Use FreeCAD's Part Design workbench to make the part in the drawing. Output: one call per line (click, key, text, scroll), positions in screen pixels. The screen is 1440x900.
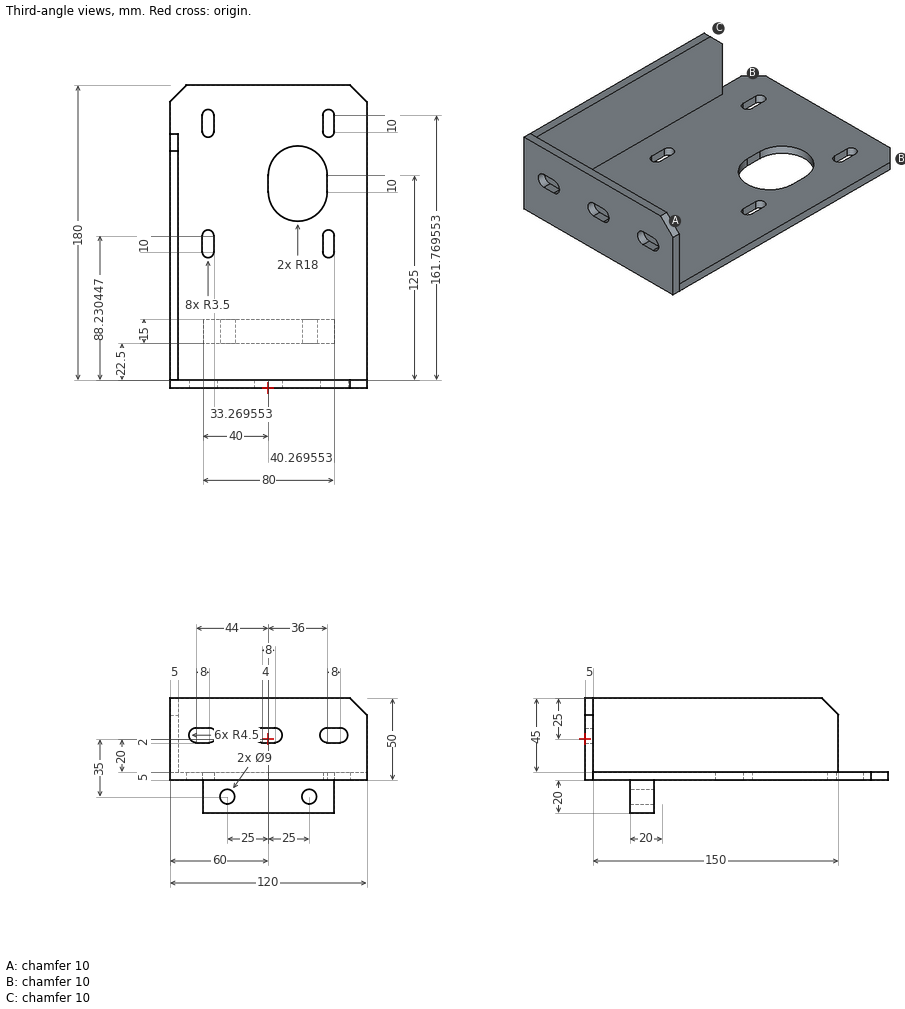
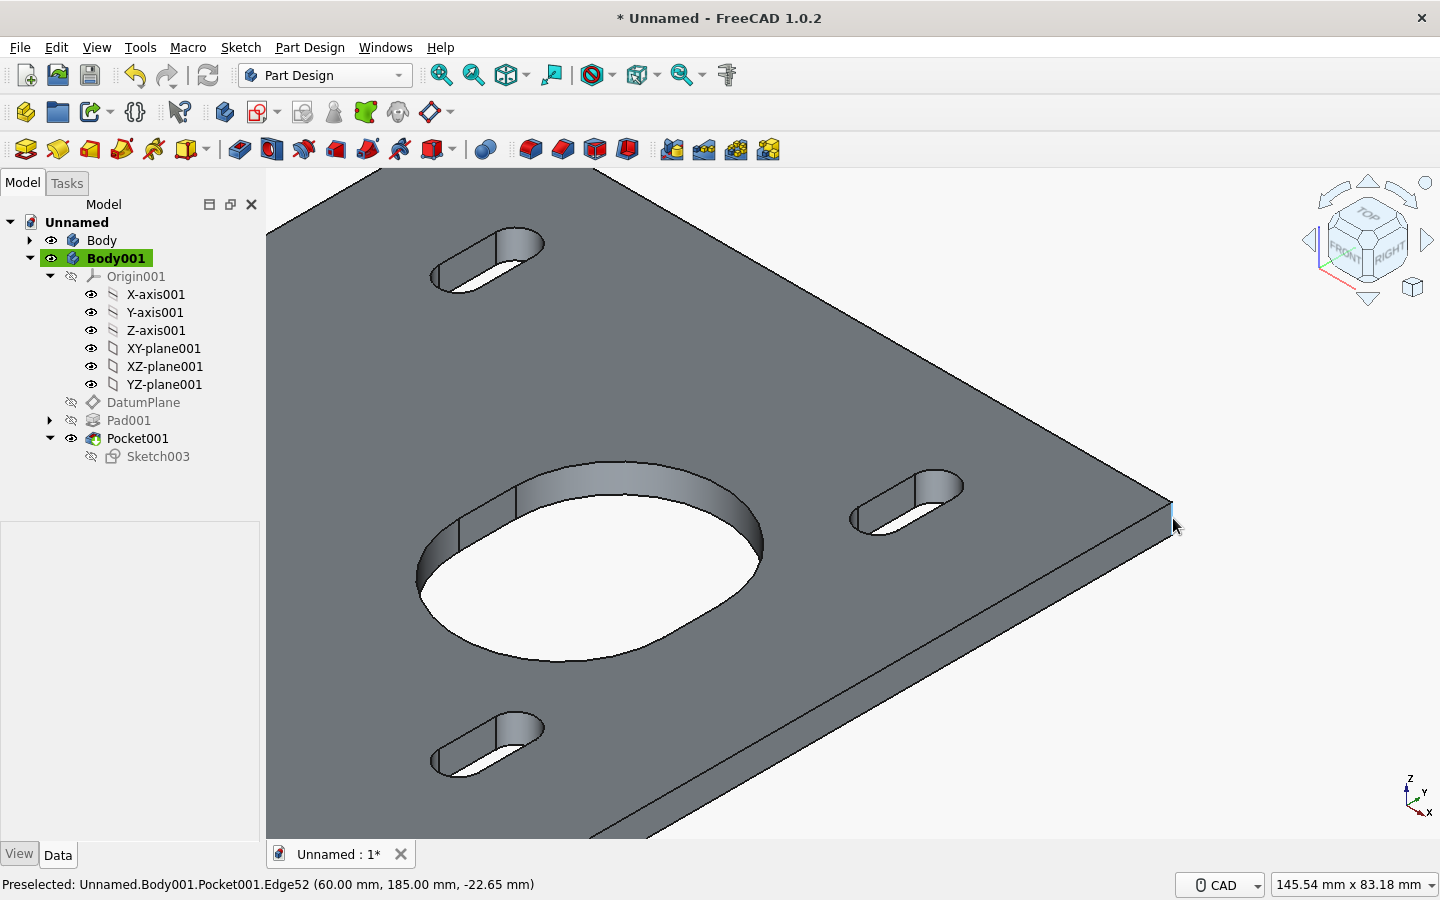
click(442, 76)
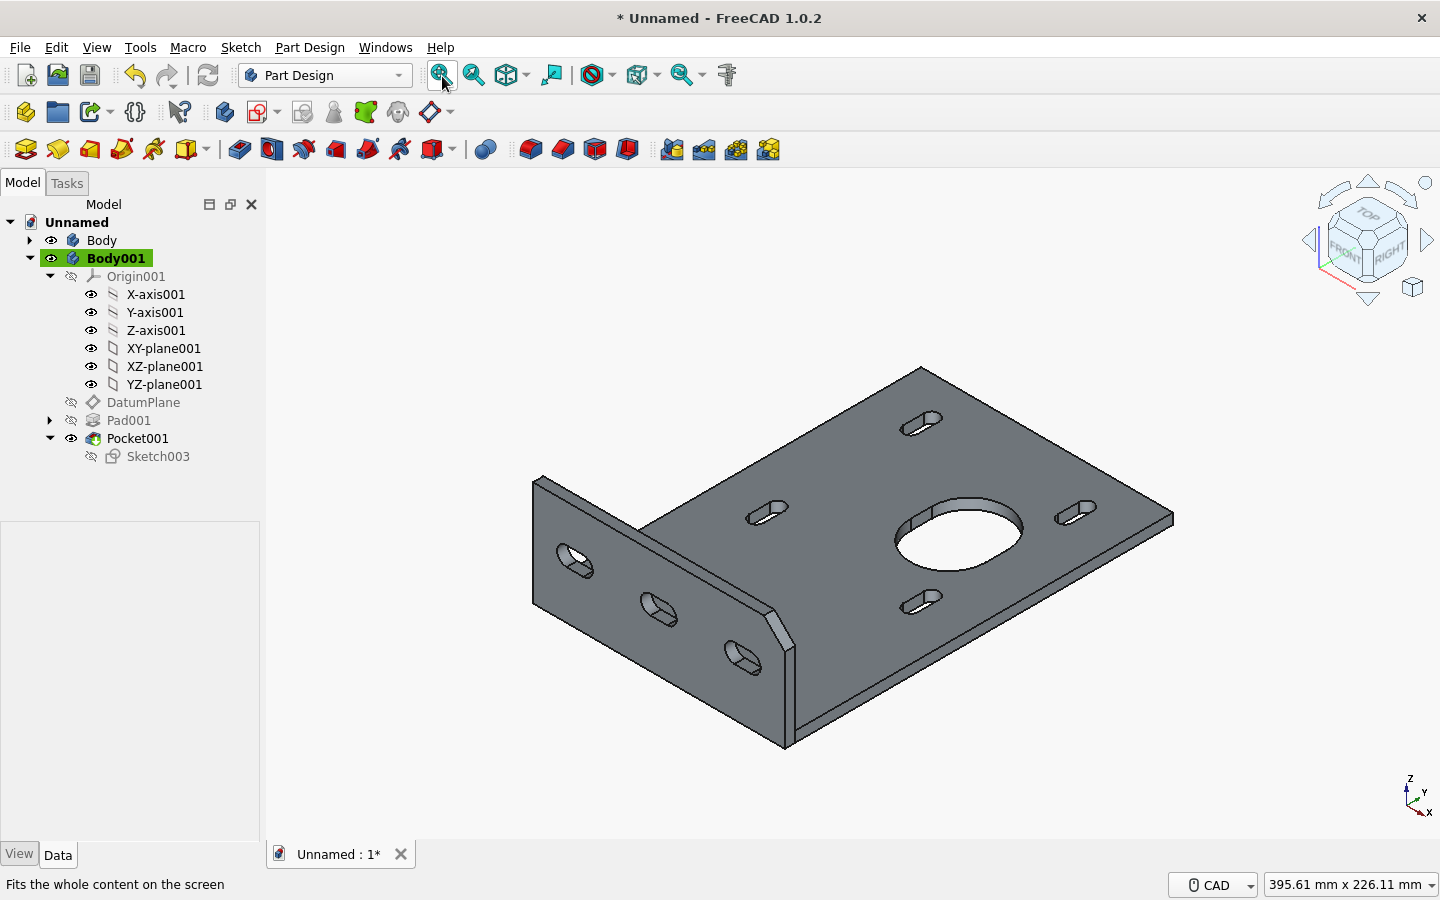
key(2)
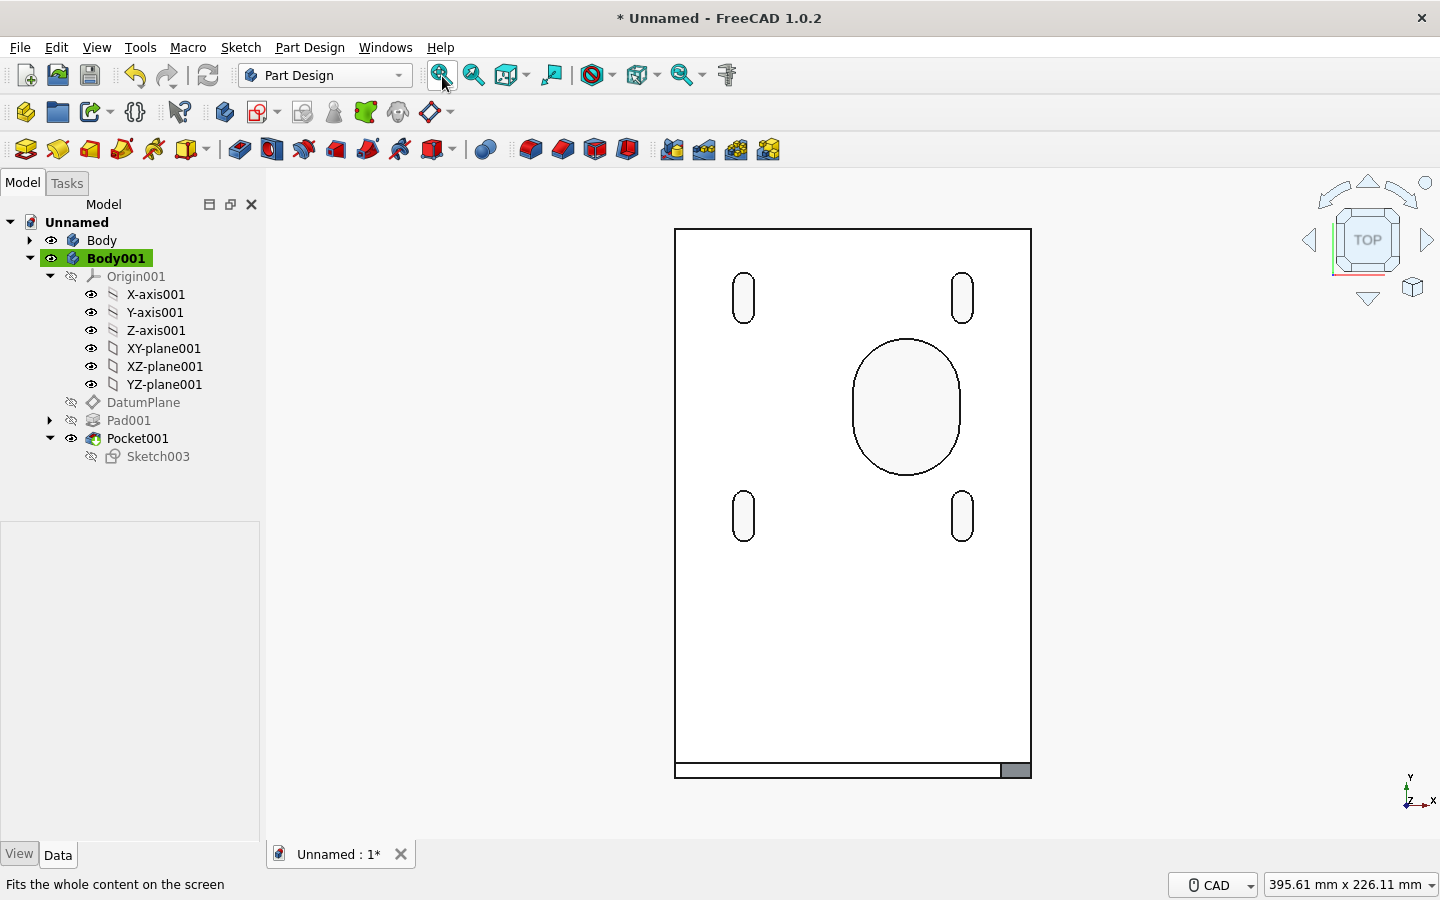
scroll(1031, 228, up, 5)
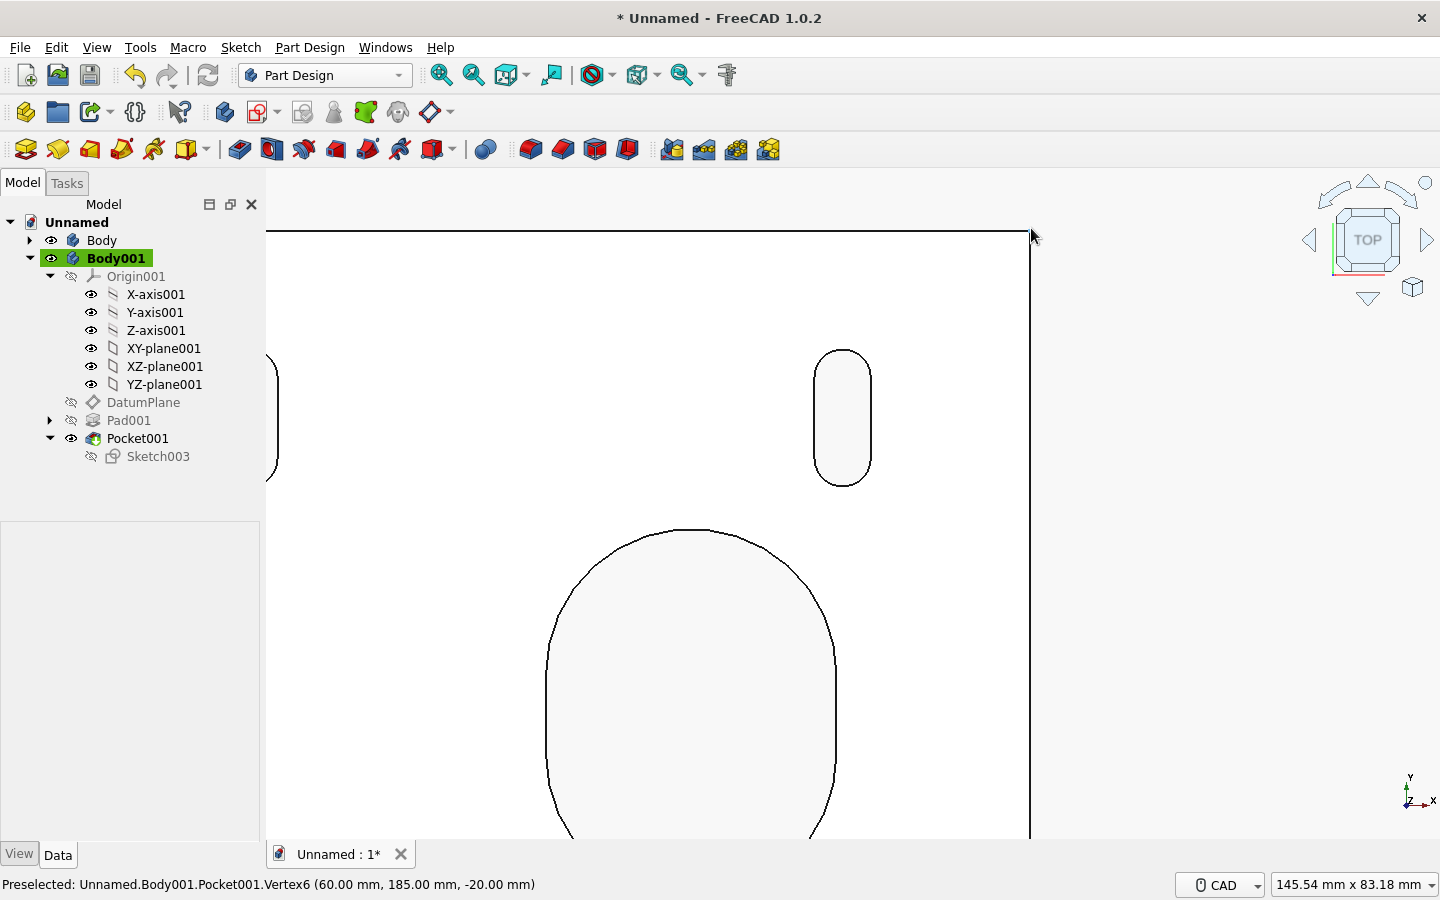
key(v)
key(f)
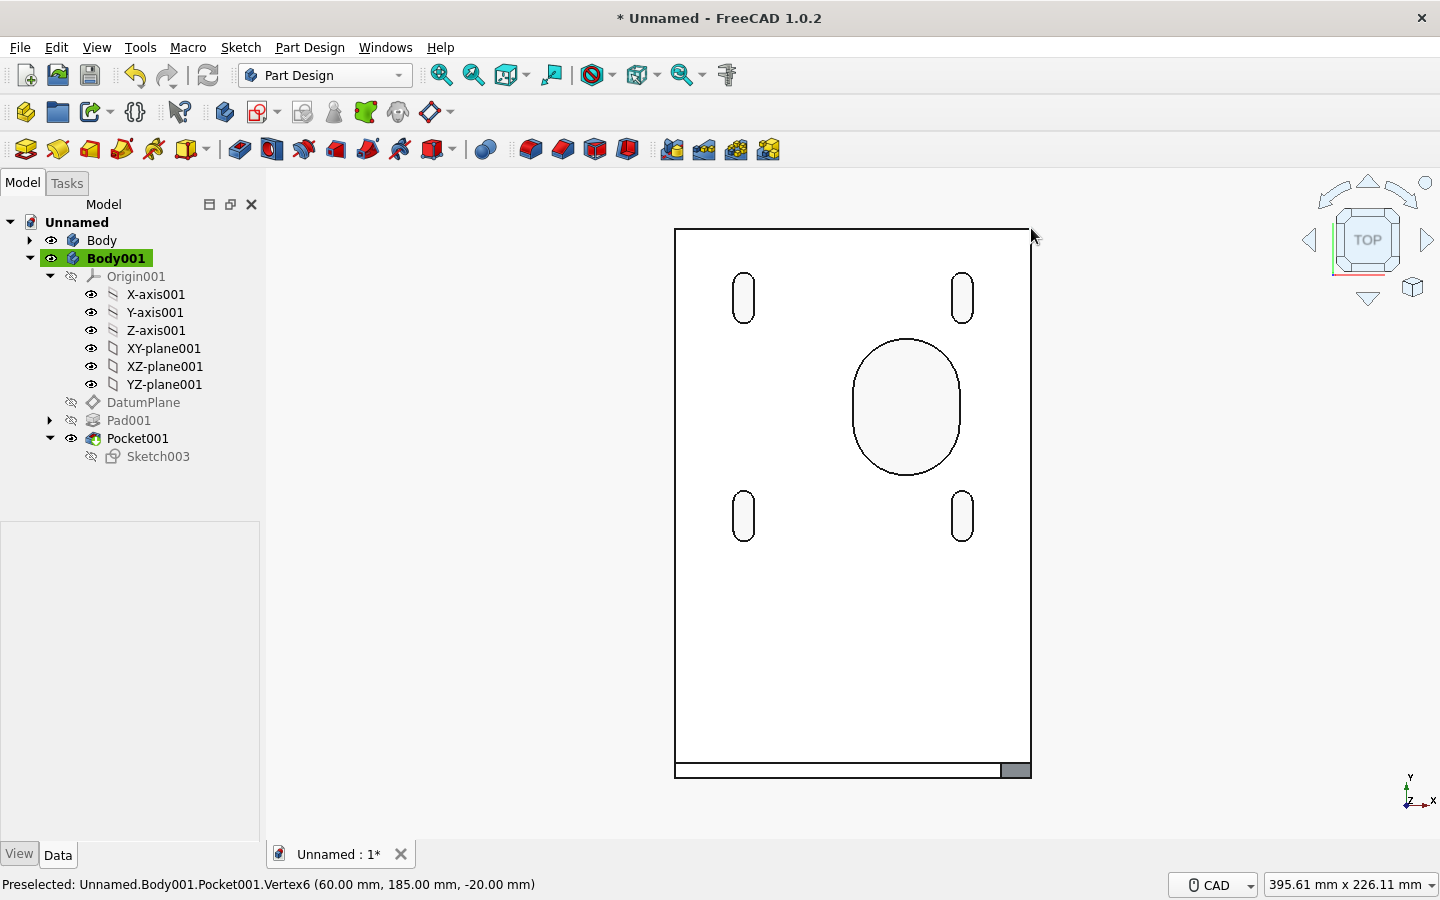
key(0)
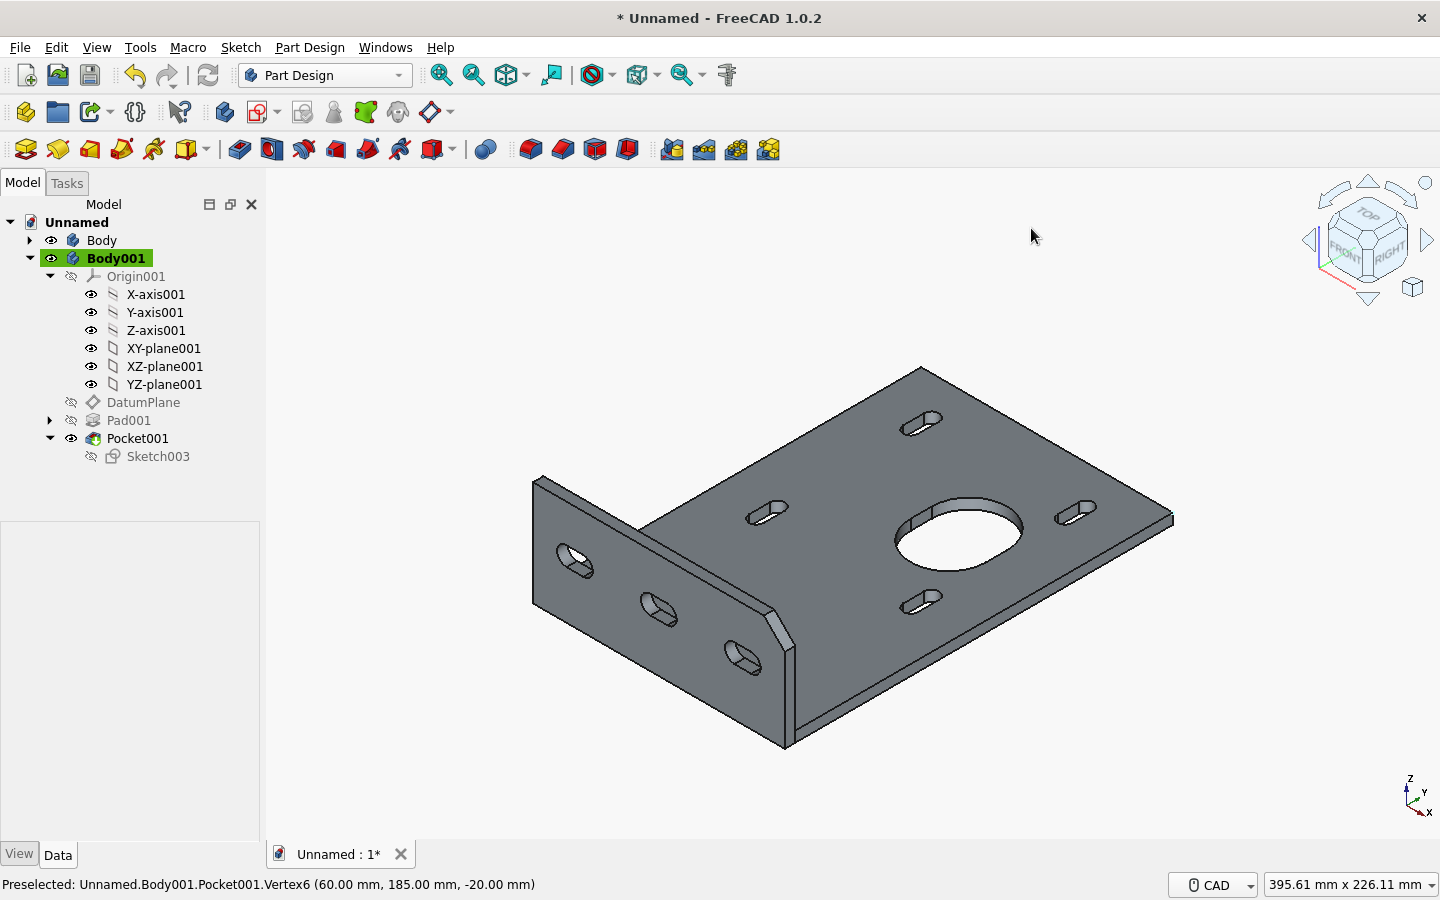
scroll(1173, 518, up, 5)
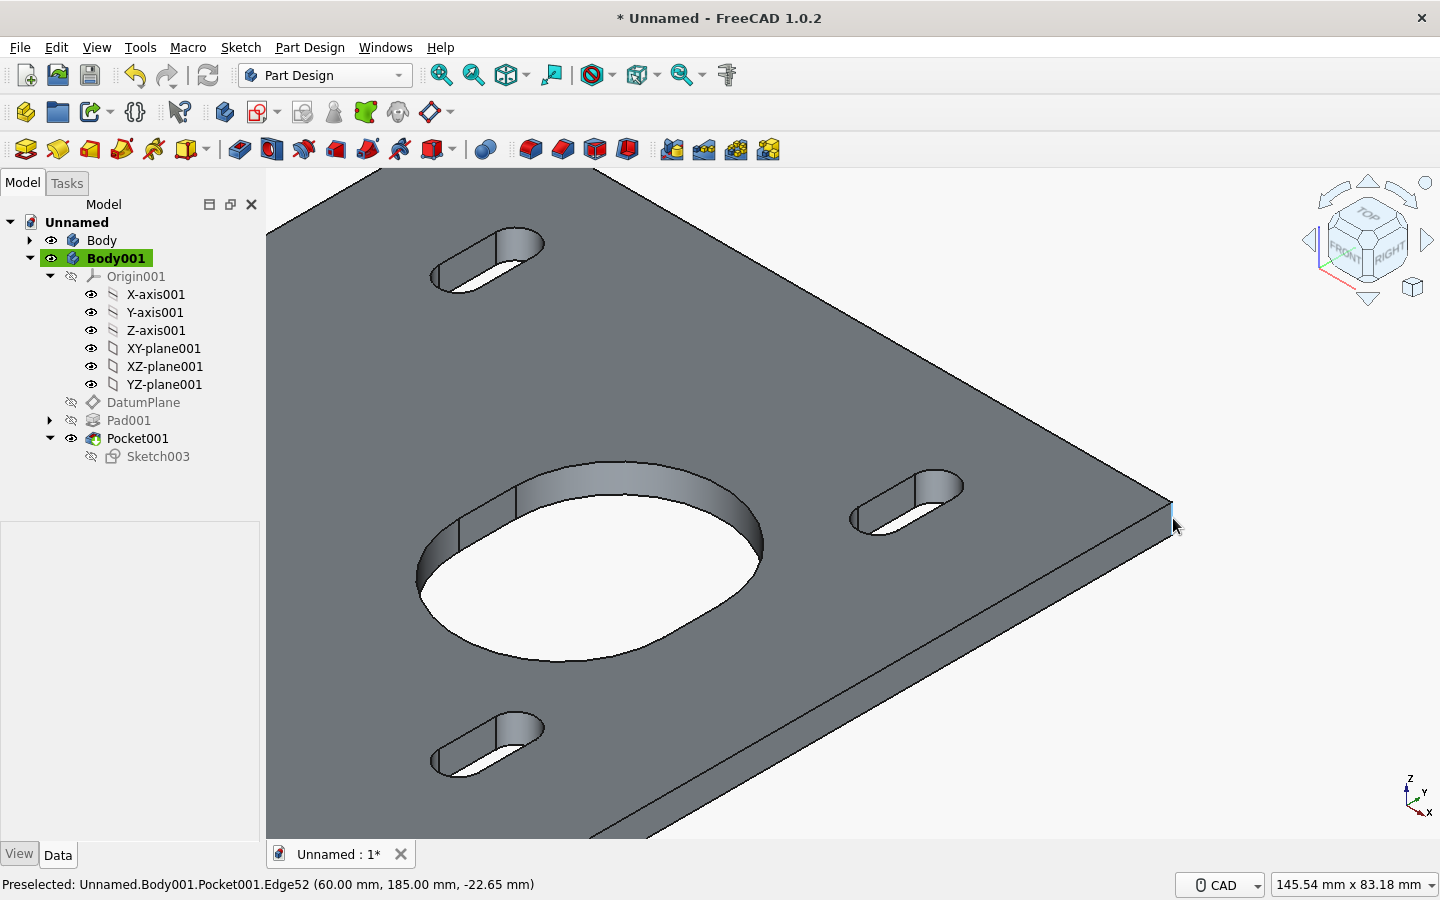
key(v)
key(f)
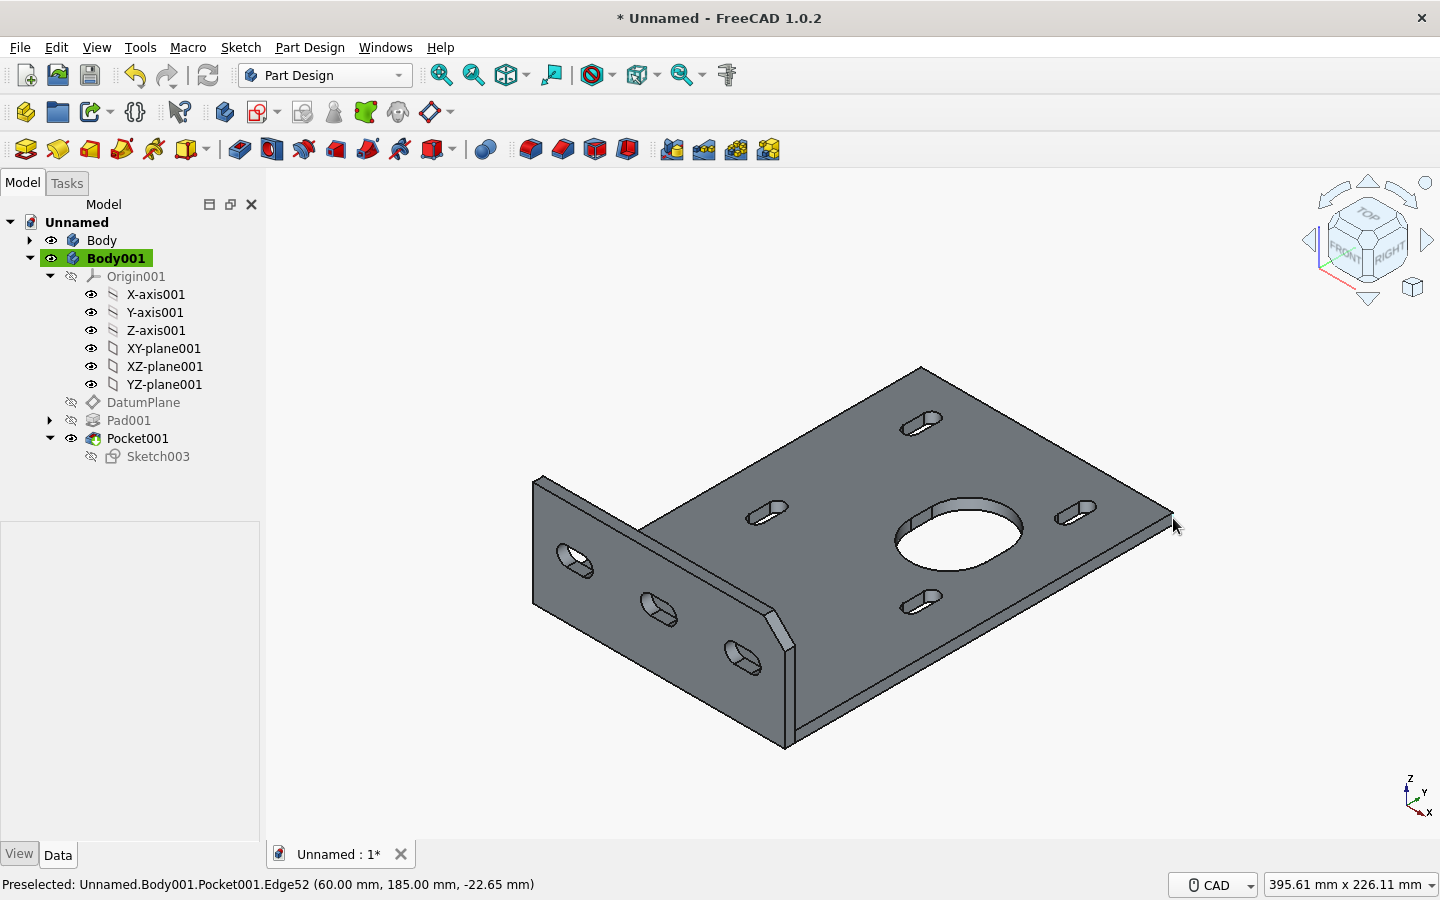
key(1)